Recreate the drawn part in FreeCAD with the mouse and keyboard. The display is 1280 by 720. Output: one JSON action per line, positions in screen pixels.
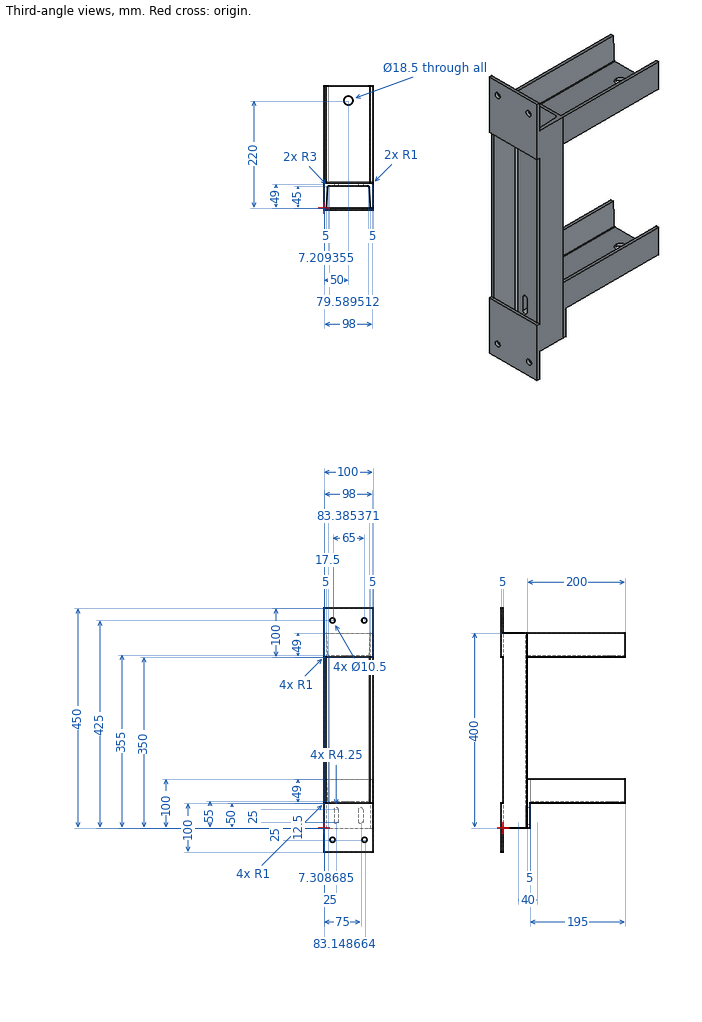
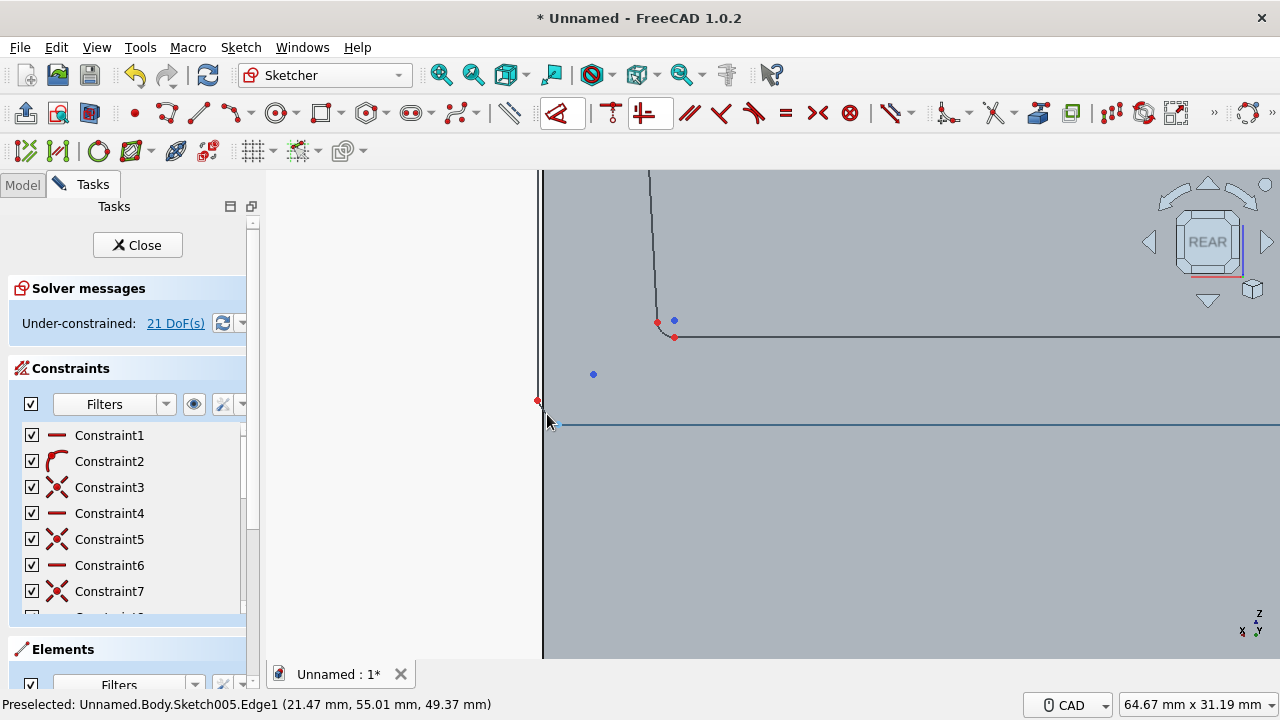
{"action": "left_click", "coordinate": [546, 414]}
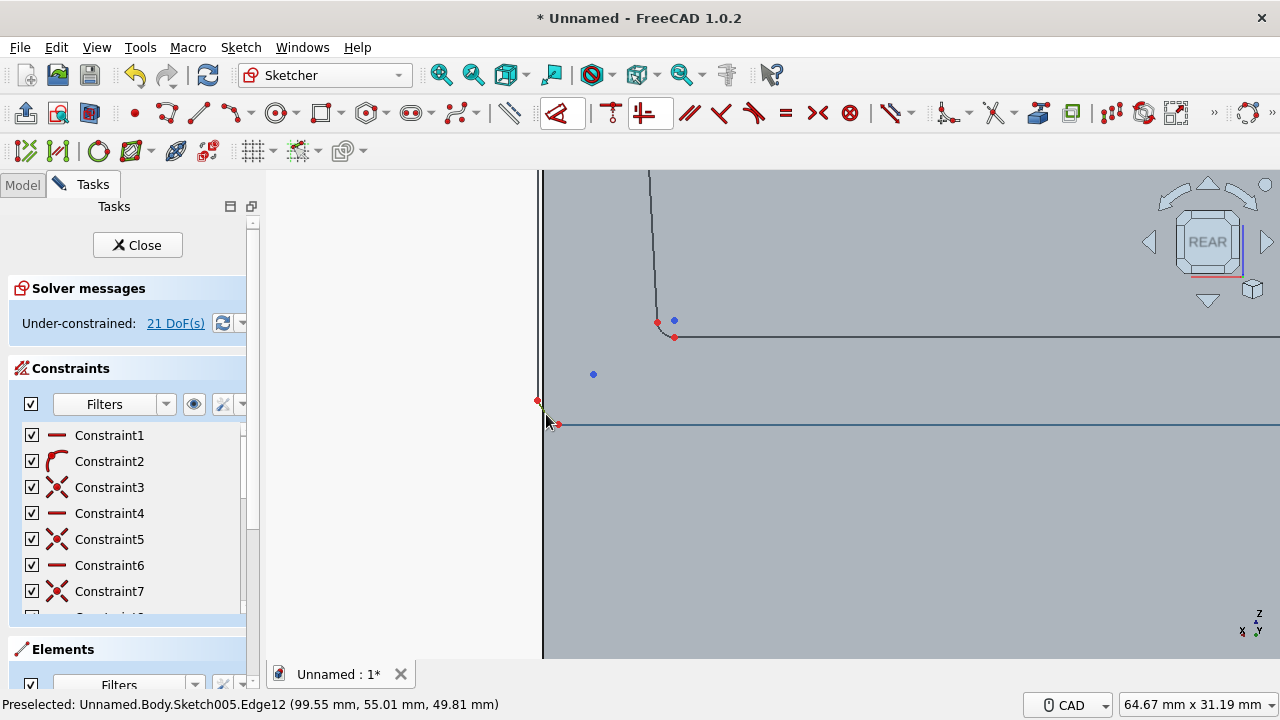
{"action": "left_click", "coordinate": [754, 114]}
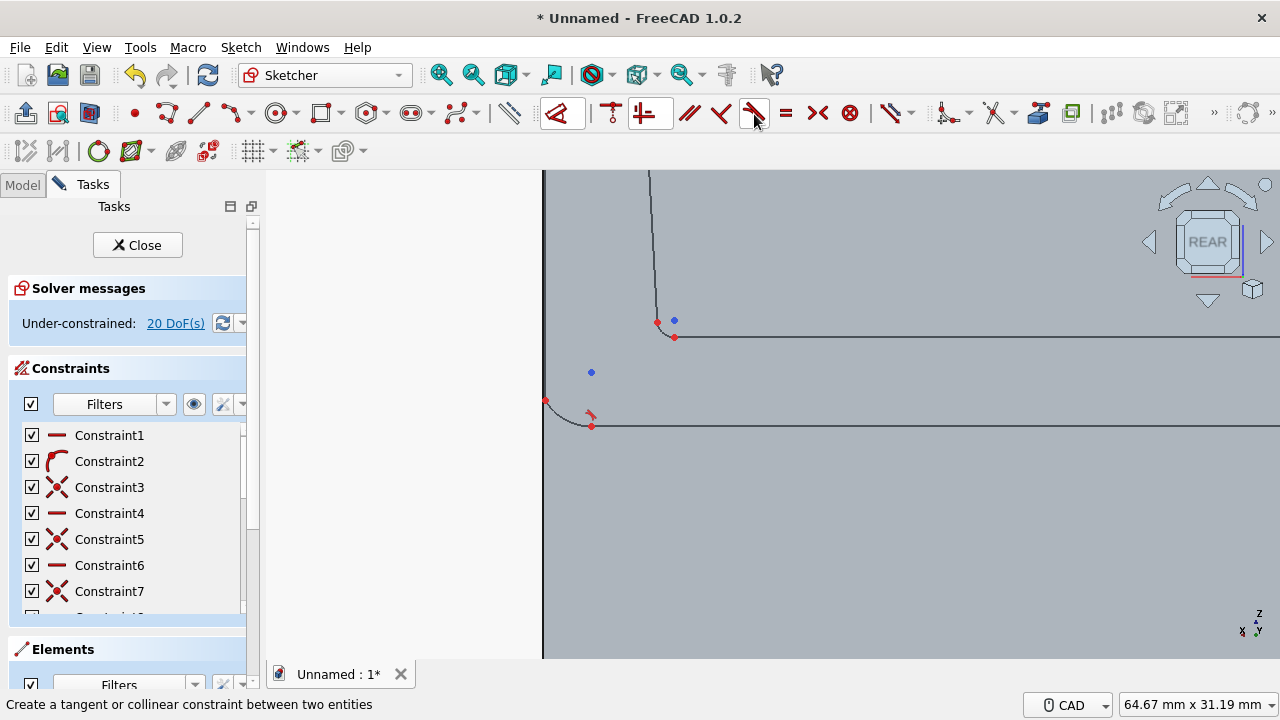
{"action": "scroll", "coordinate": [547, 414], "scroll_direction": "down", "scroll_amount": 8}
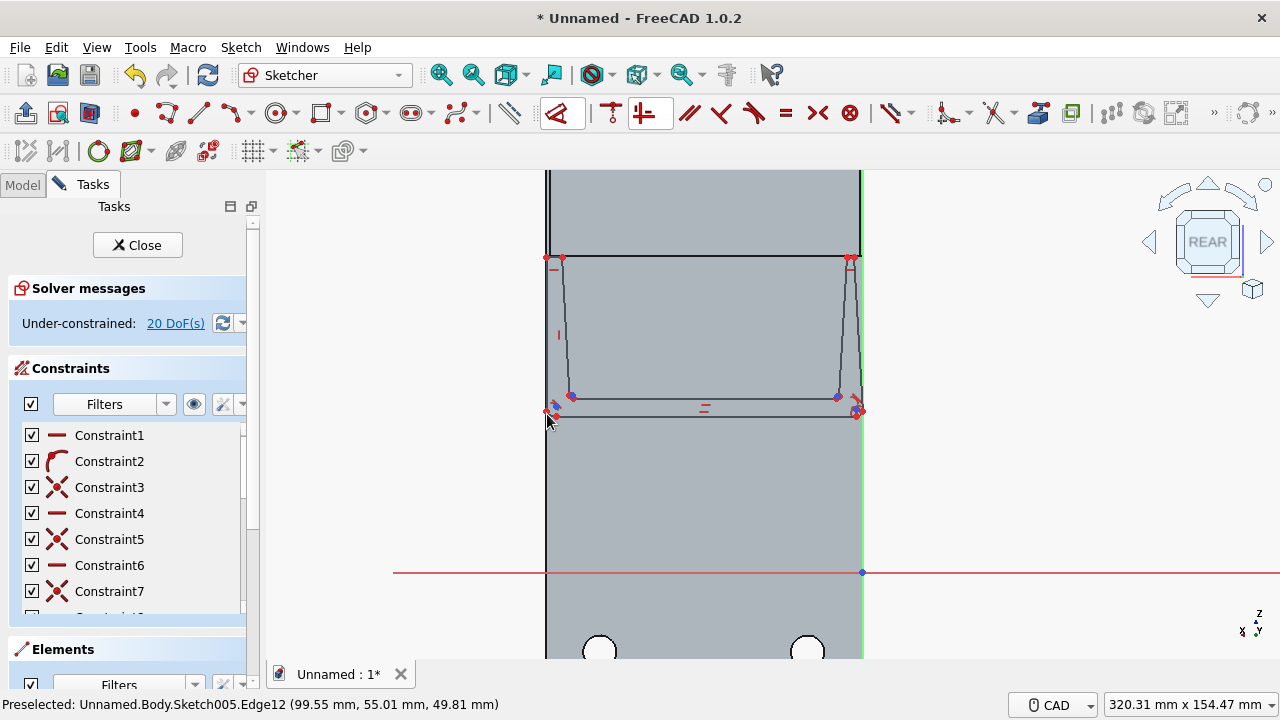
{"action": "scroll", "coordinate": [860, 365], "scroll_direction": "up", "scroll_amount": 9}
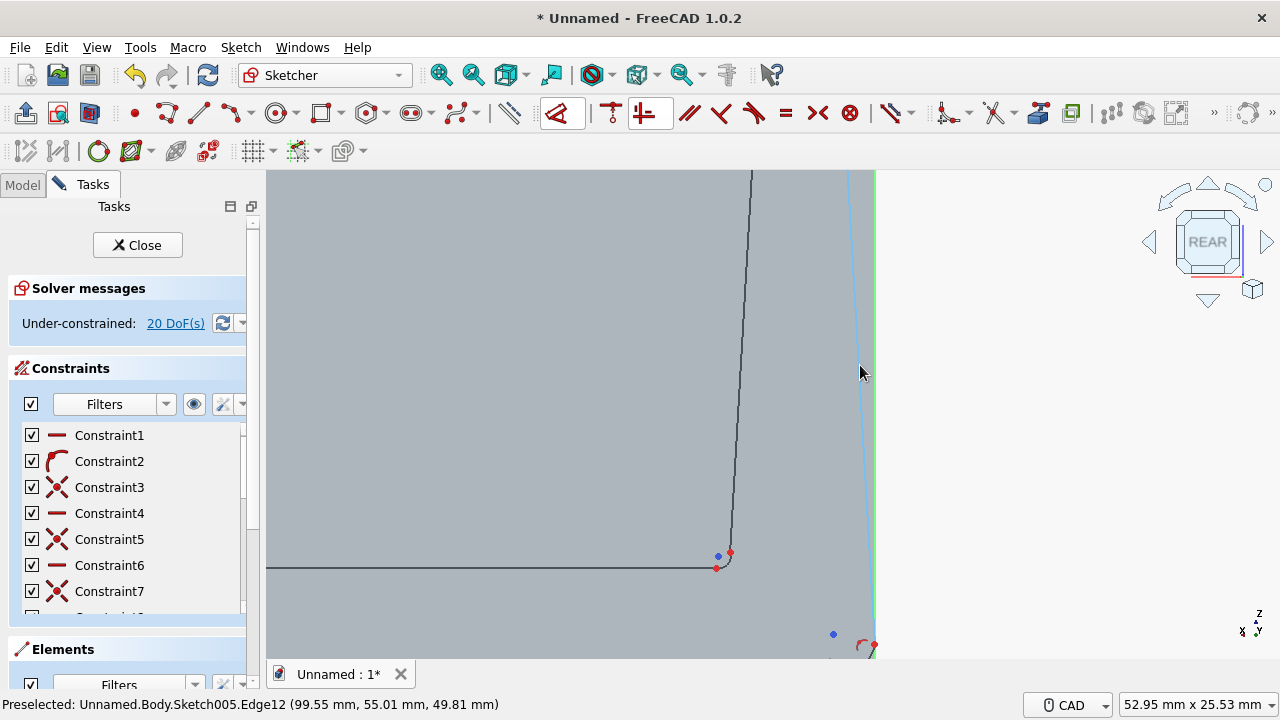
{"action": "left_click", "coordinate": [859, 365]}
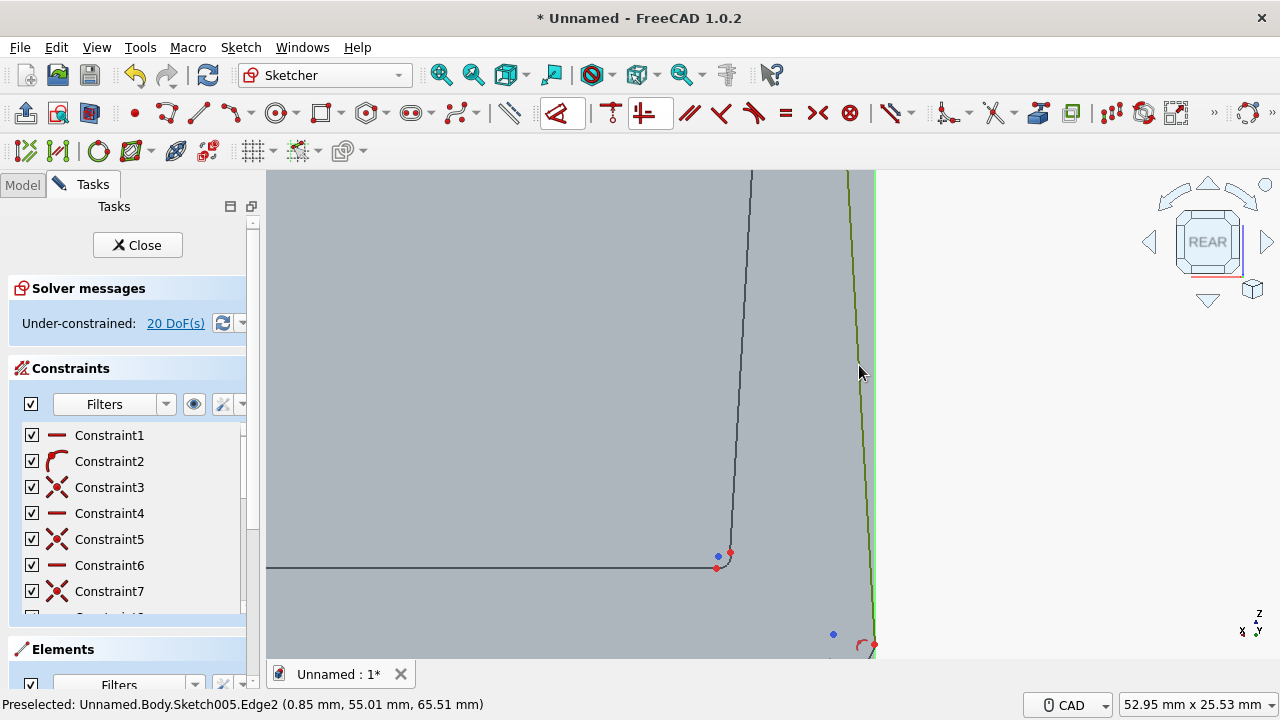
{"action": "scroll", "coordinate": [860, 365], "scroll_direction": "down", "scroll_amount": 9}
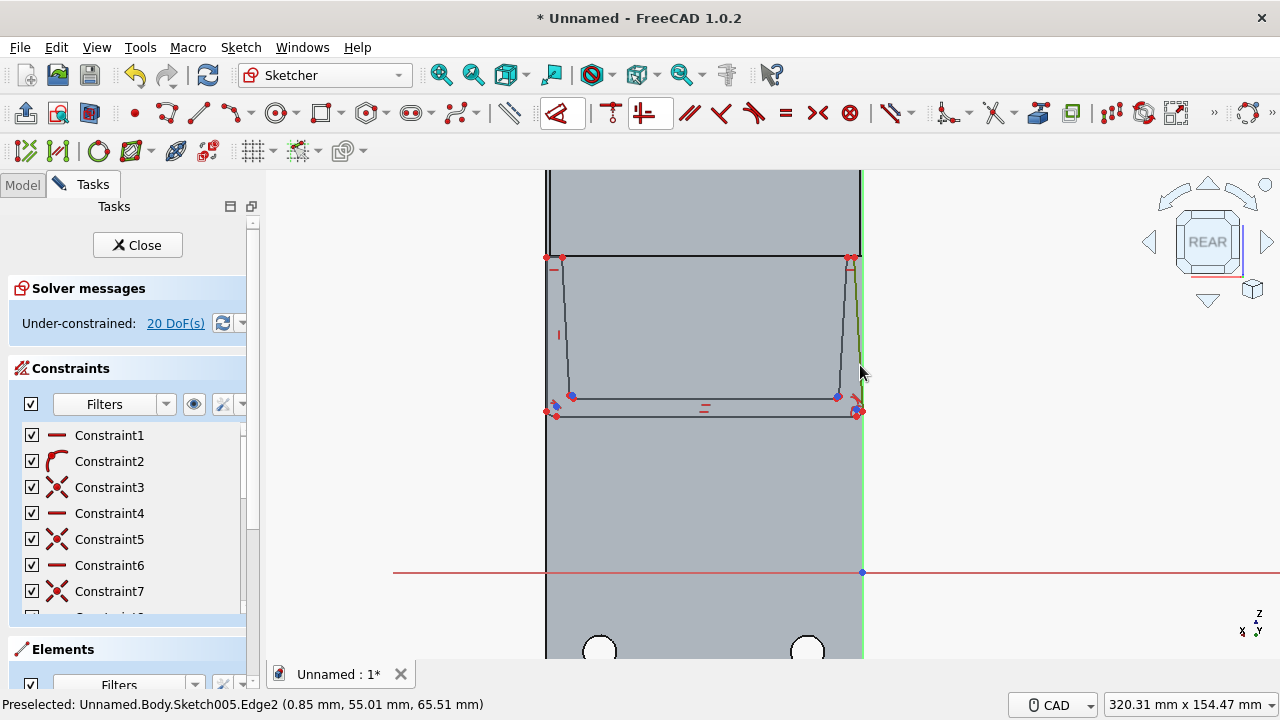
{"action": "scroll", "coordinate": [859, 416], "scroll_direction": "up", "scroll_amount": 9}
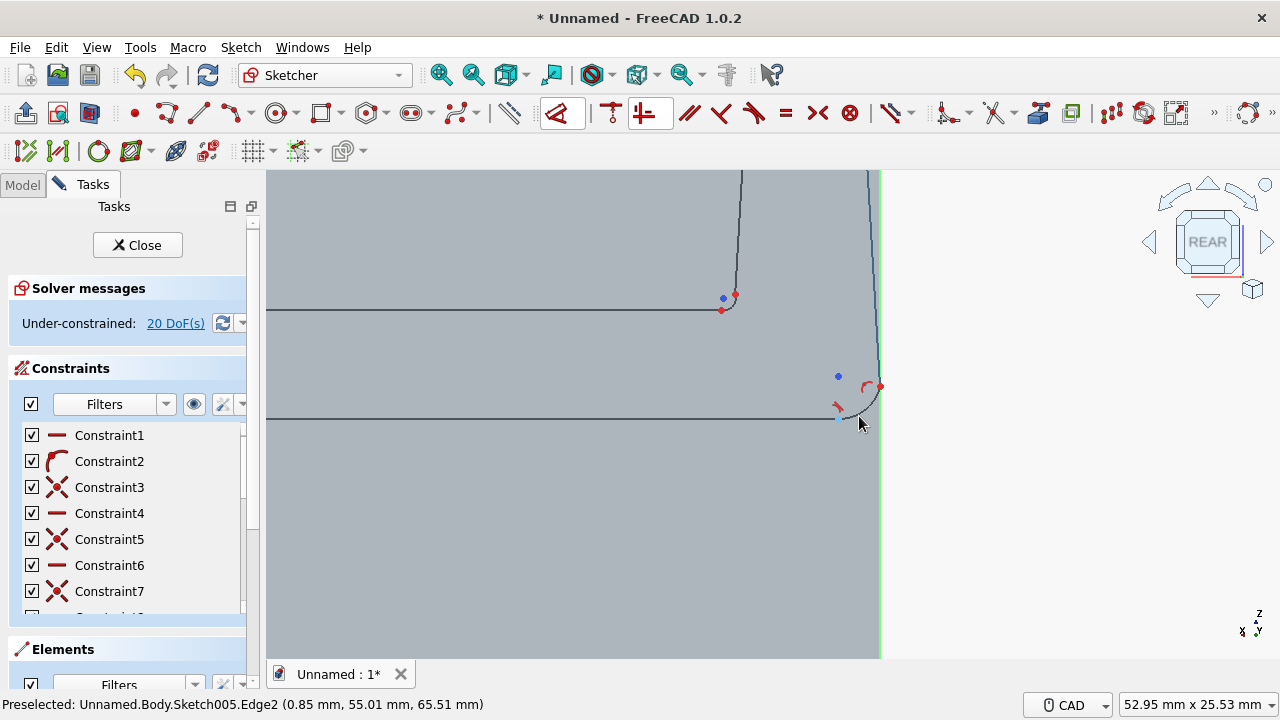
{"action": "left_click", "coordinate": [855, 416]}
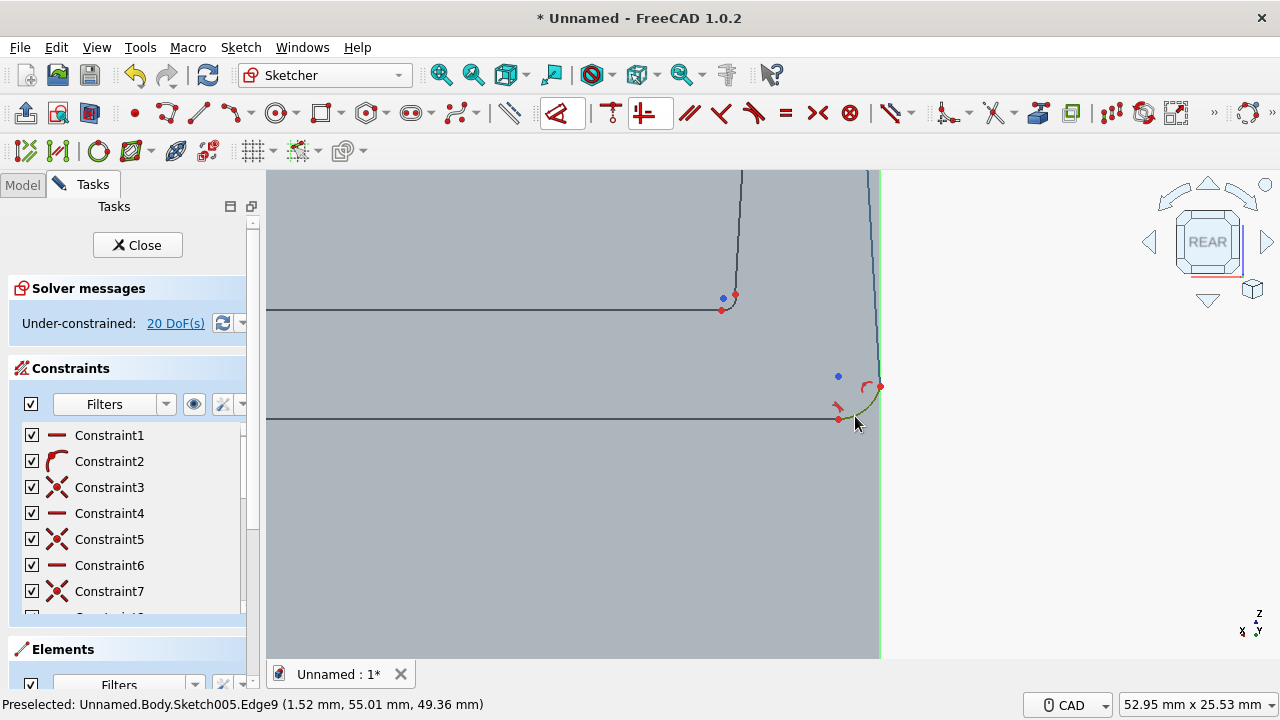
{"action": "left_click", "coordinate": [754, 114]}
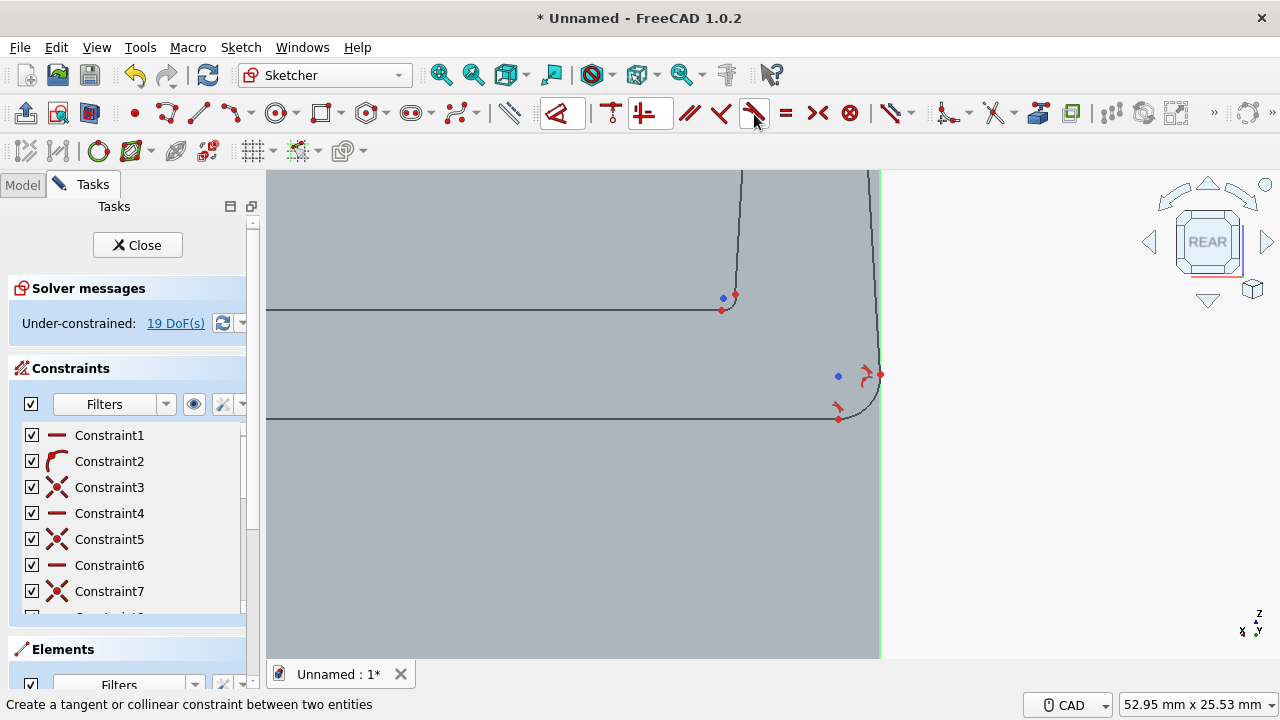
{"action": "scroll", "coordinate": [859, 416], "scroll_direction": "down", "scroll_amount": 9}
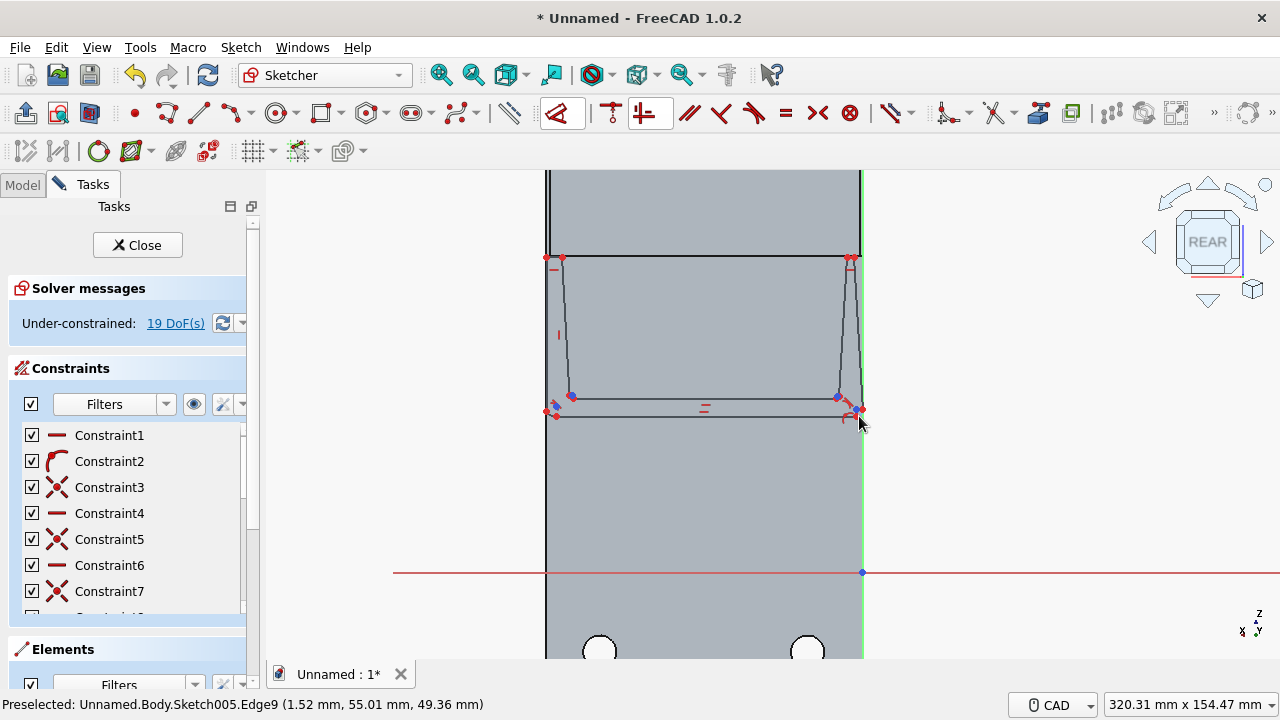
{"action": "left_click", "coordinate": [845, 299]}